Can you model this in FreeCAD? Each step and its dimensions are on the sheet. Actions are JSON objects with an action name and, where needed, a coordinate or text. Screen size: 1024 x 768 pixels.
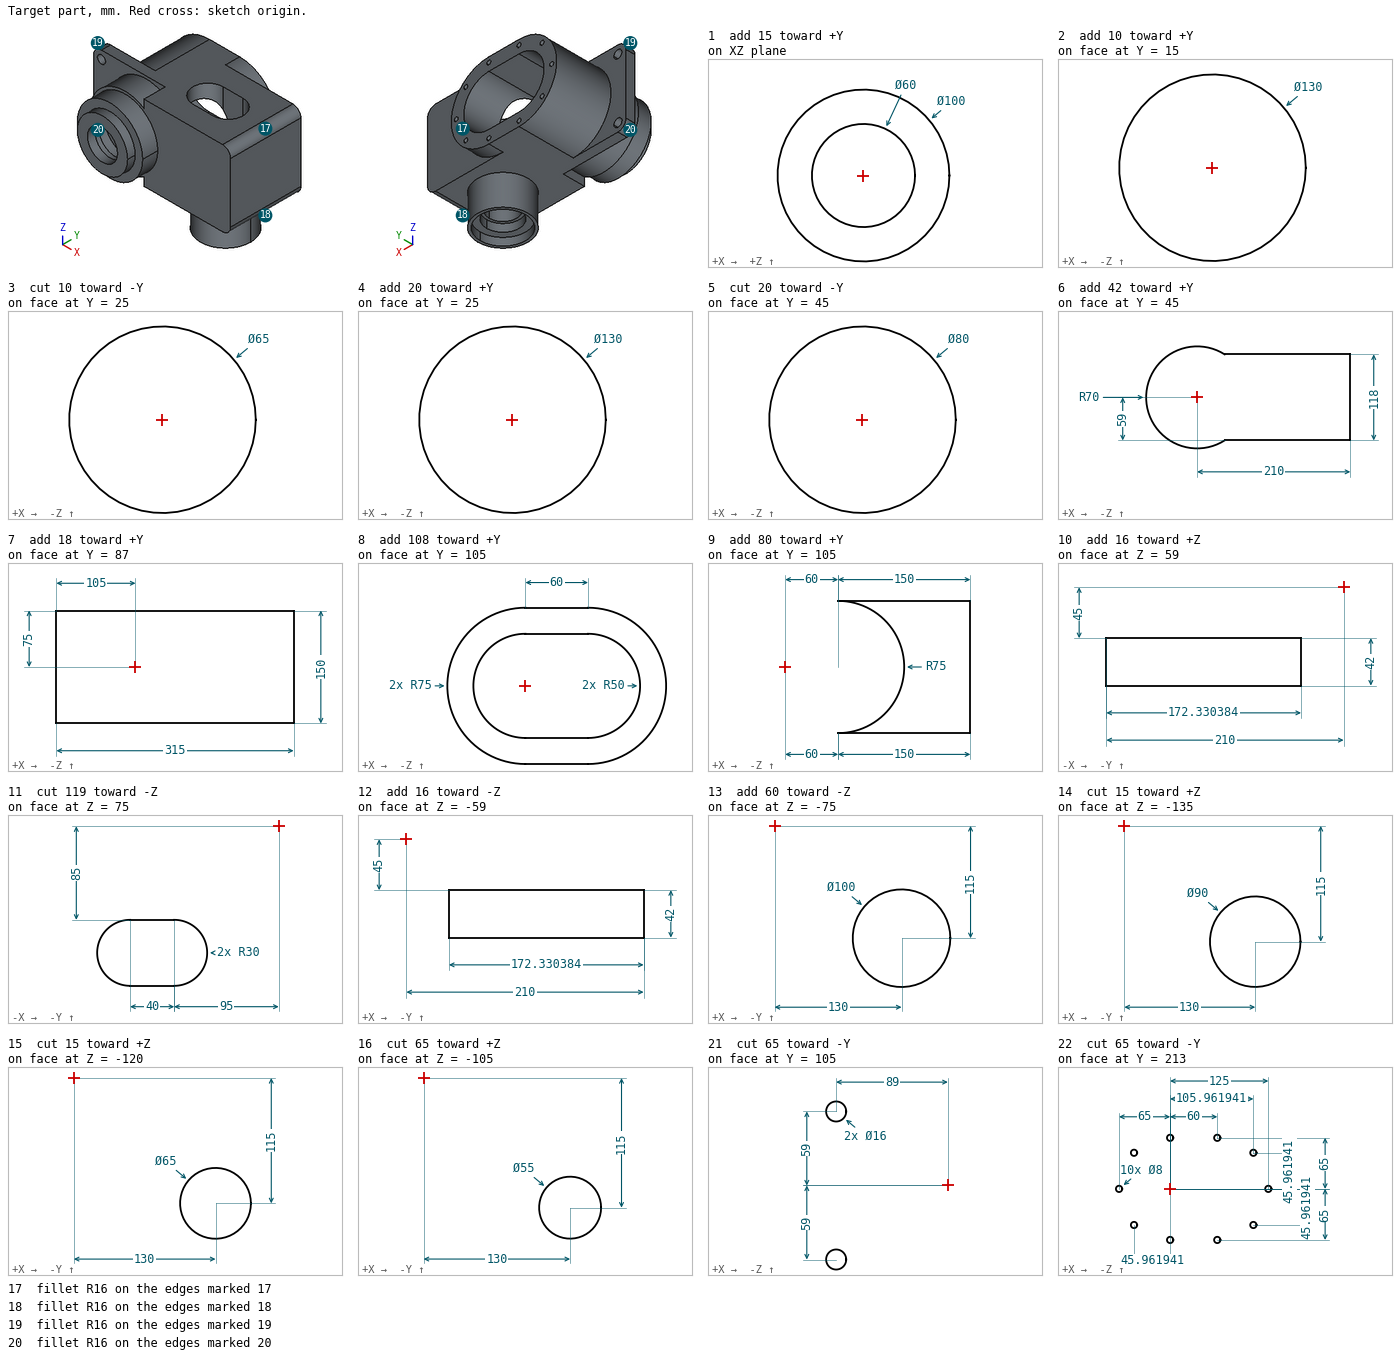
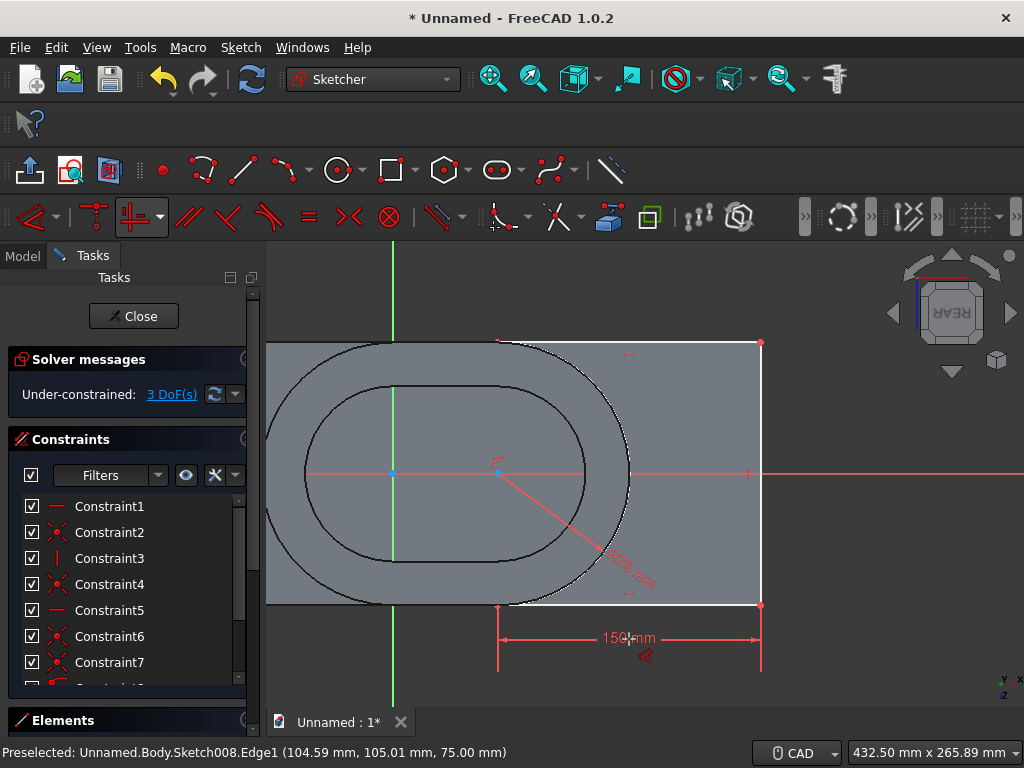
{"action": "left_click", "coordinate": [682, 342]}
{"action": "left_click", "coordinate": [629, 308]}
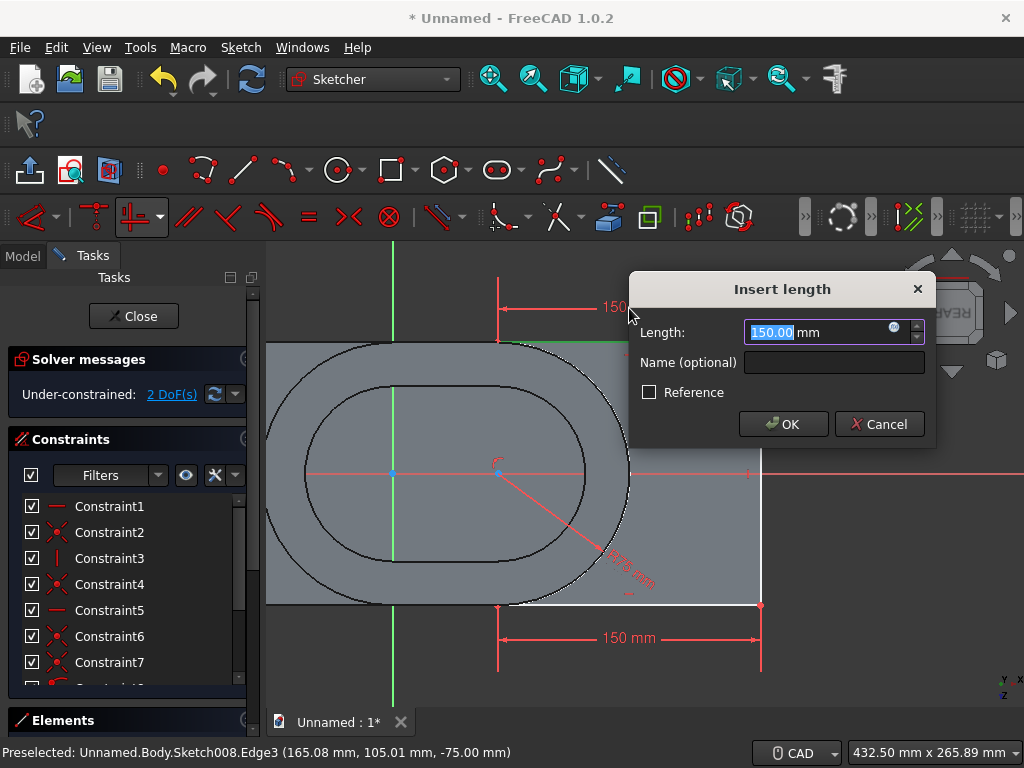
{"action": "type", "text": "150"}
{"action": "key", "text": "Return"}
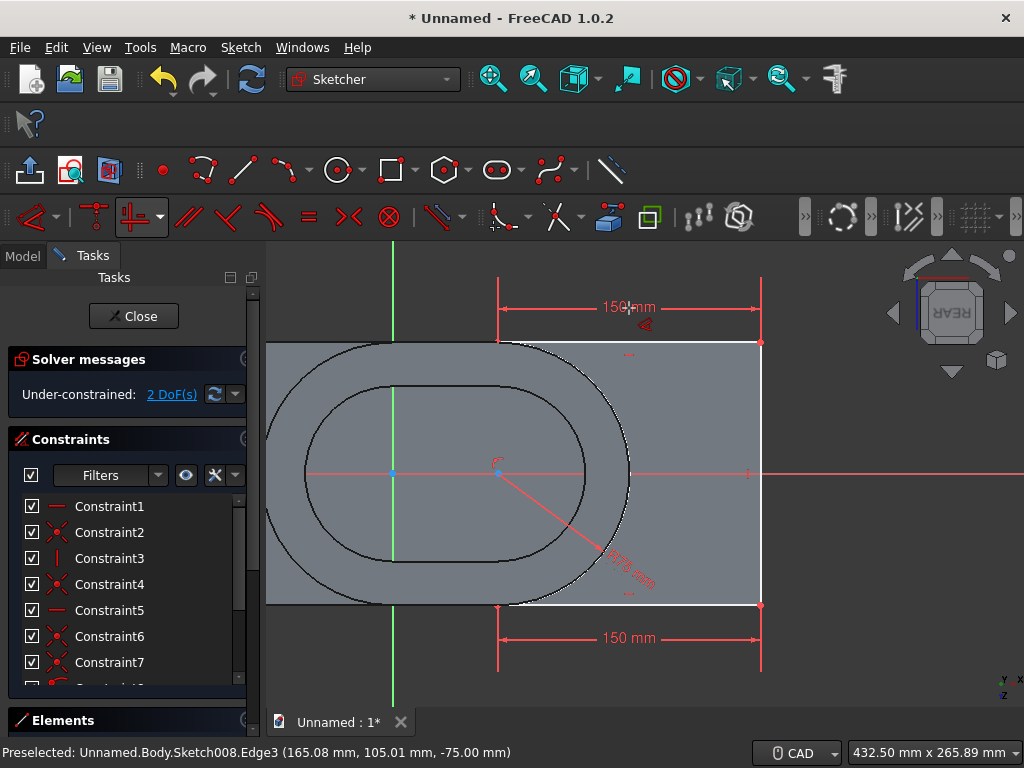
{"action": "left_click", "coordinate": [498, 605]}
{"action": "left_click", "coordinate": [445, 639]}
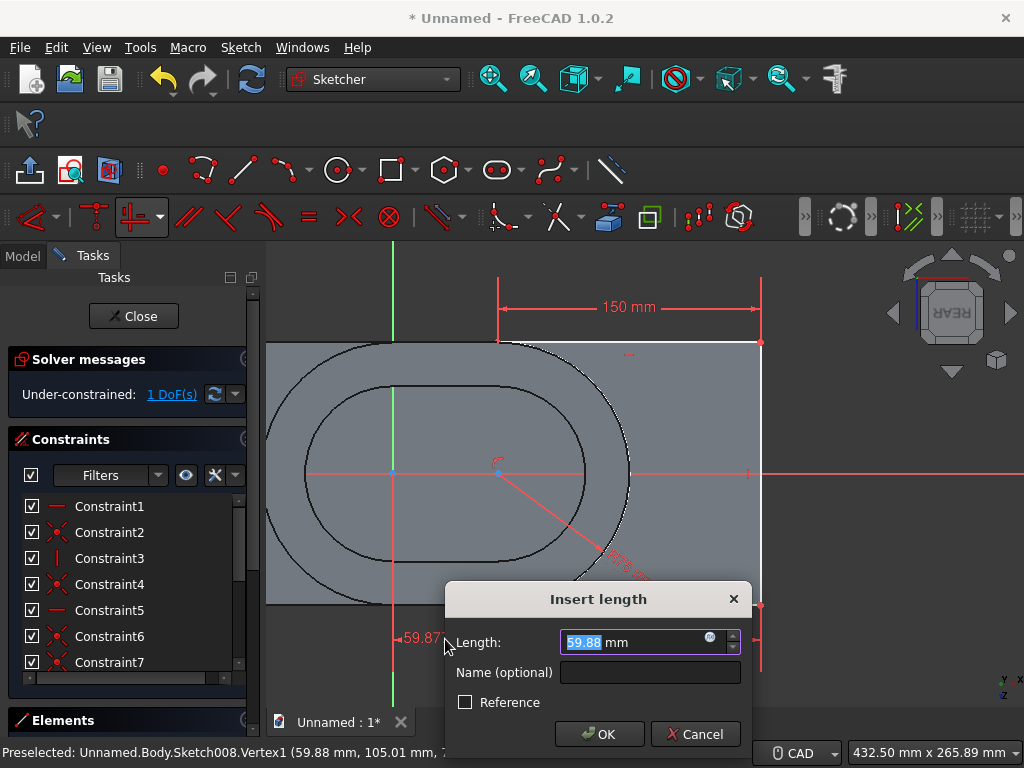
{"action": "type", "text": "60"}
{"action": "key", "text": "Return"}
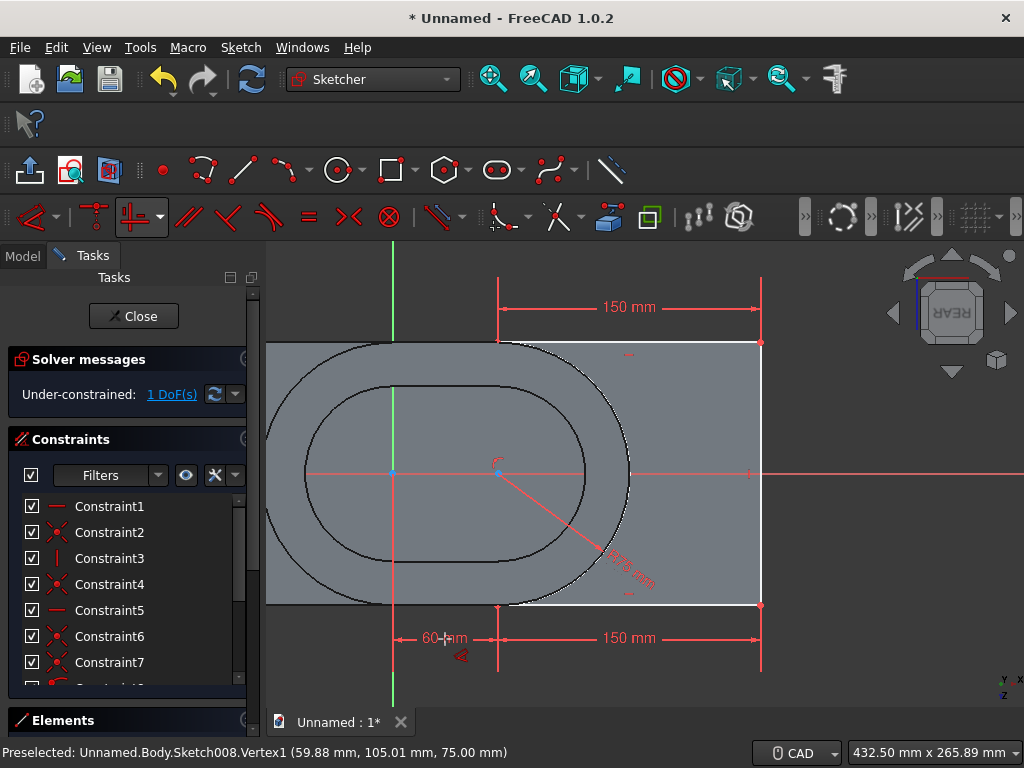
{"action": "left_click", "coordinate": [498, 474]}
{"action": "left_click", "coordinate": [445, 508]}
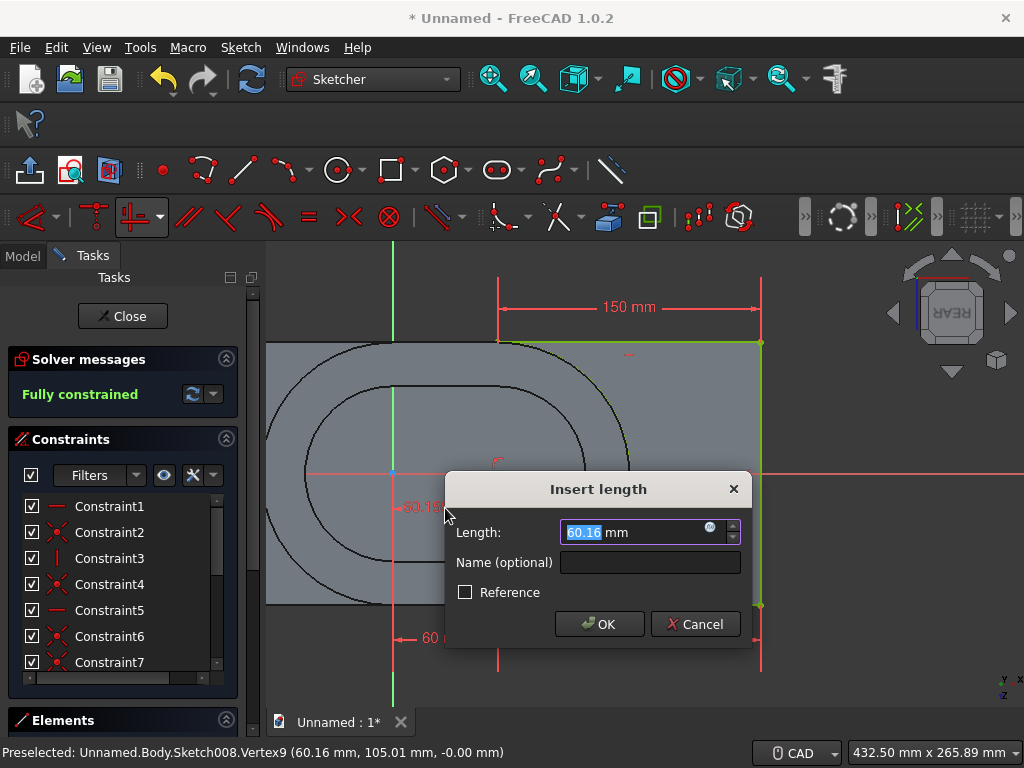
{"action": "type", "text": "60"}
{"action": "key", "text": "Return"}
{"action": "key", "text": "Escape"}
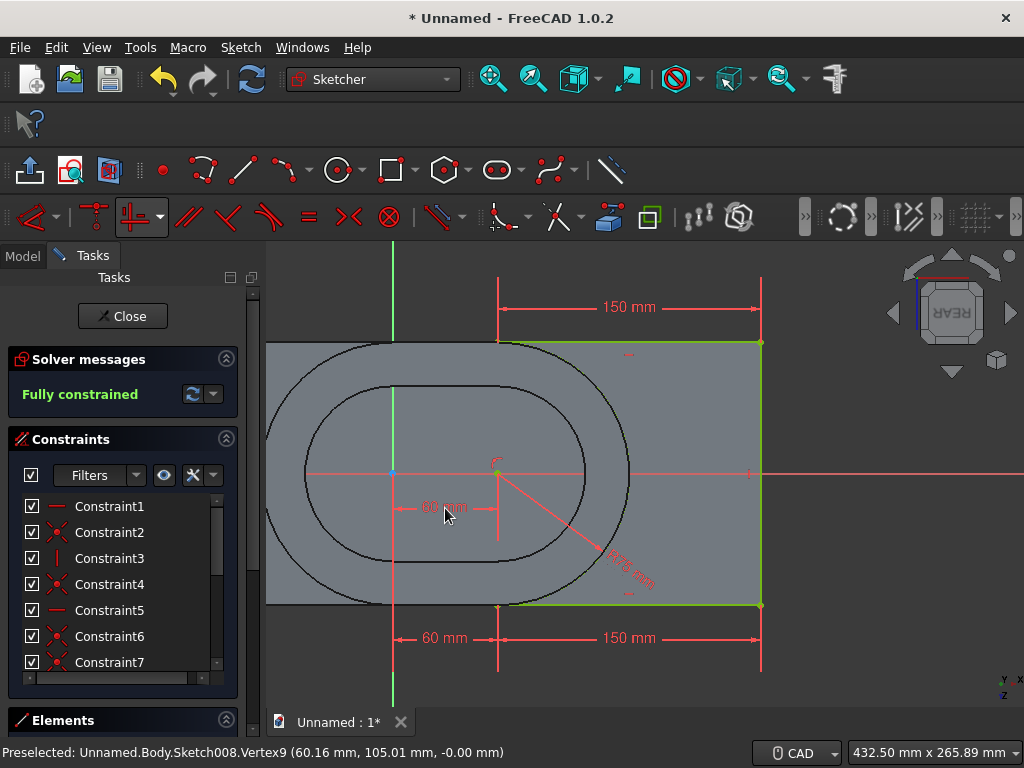
{"action": "left_click", "coordinate": [123, 316]}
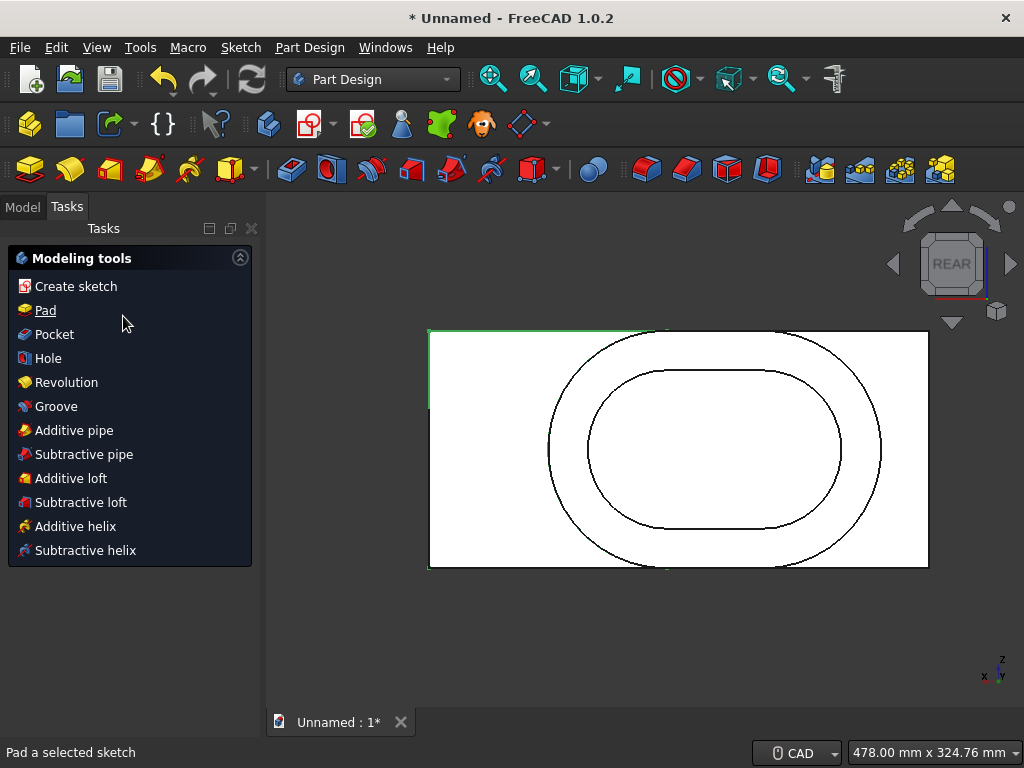
{"action": "left_click", "coordinate": [30, 170]}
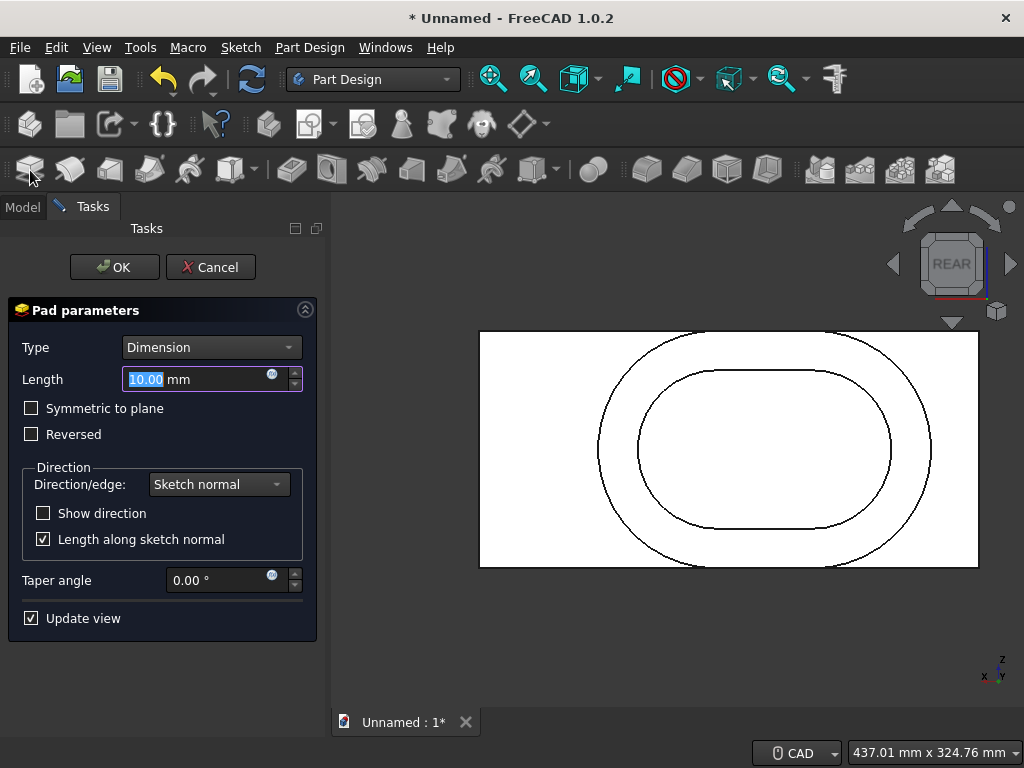
{"action": "type", "text": "80"}
{"action": "key", "text": "Tab"}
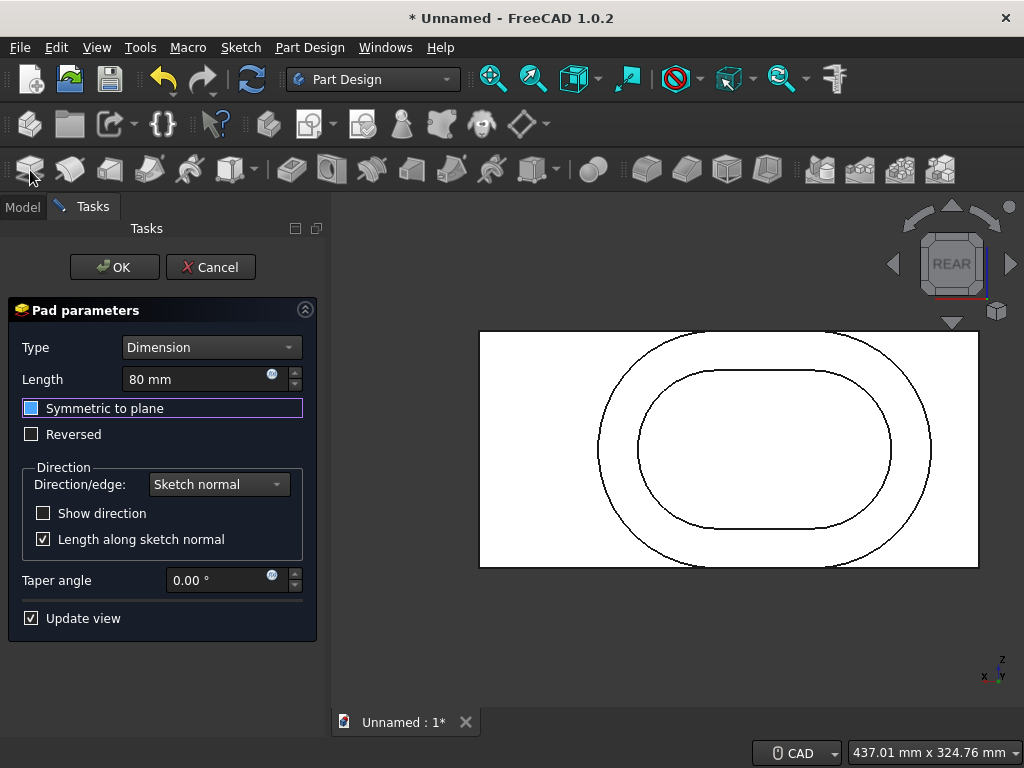
{"action": "left_click", "coordinate": [115, 267]}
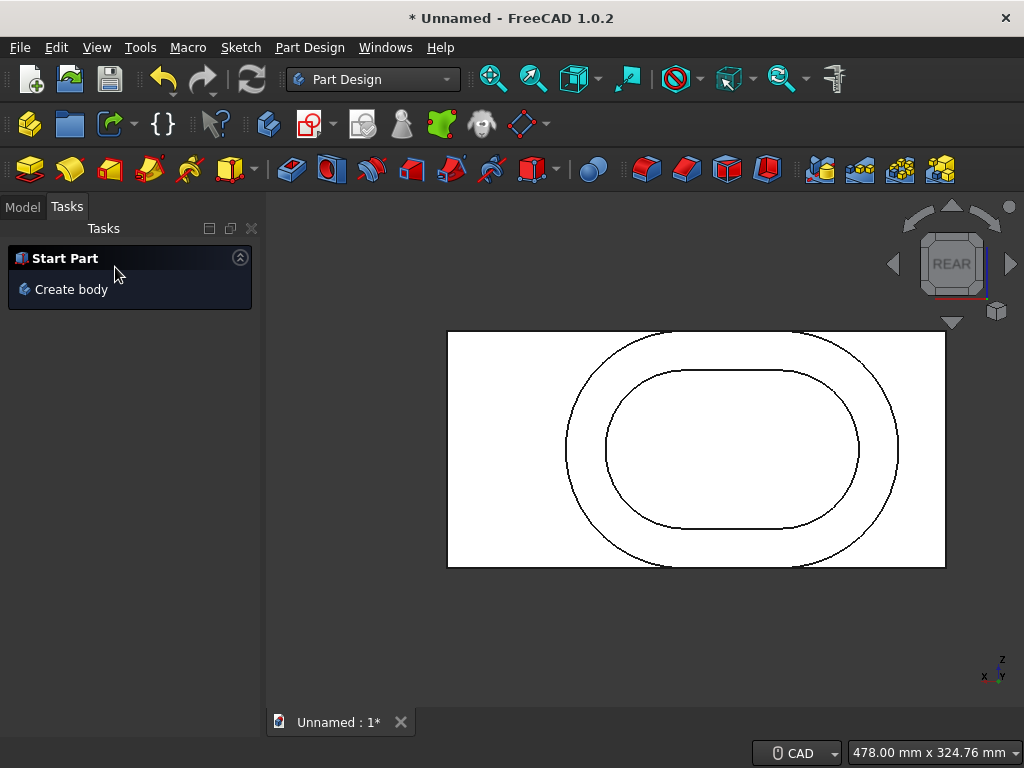
{"action": "key", "text": "0"}